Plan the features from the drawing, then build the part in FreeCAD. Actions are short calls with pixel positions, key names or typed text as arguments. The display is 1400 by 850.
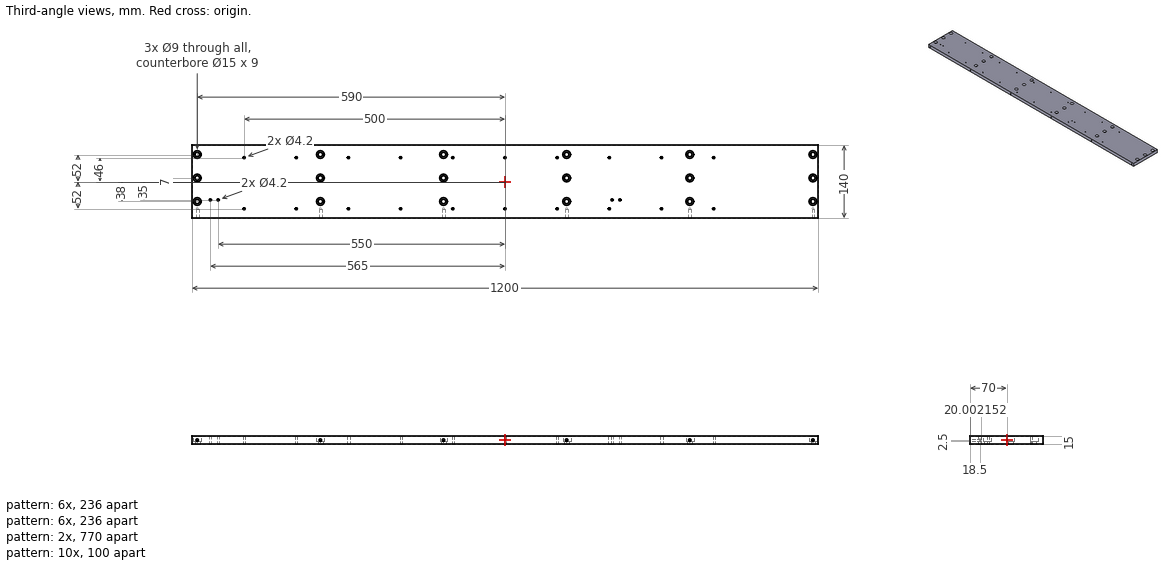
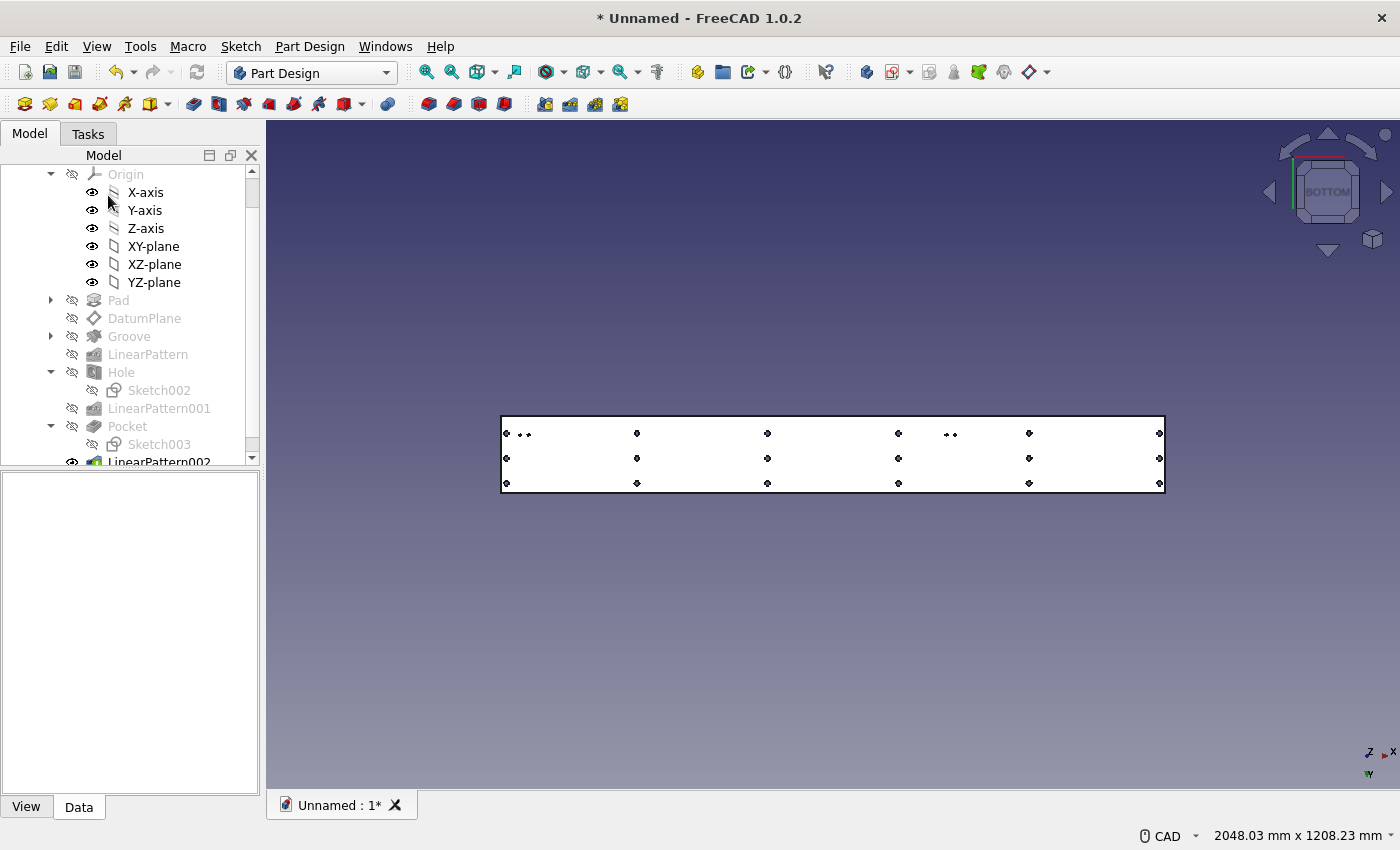
key(0)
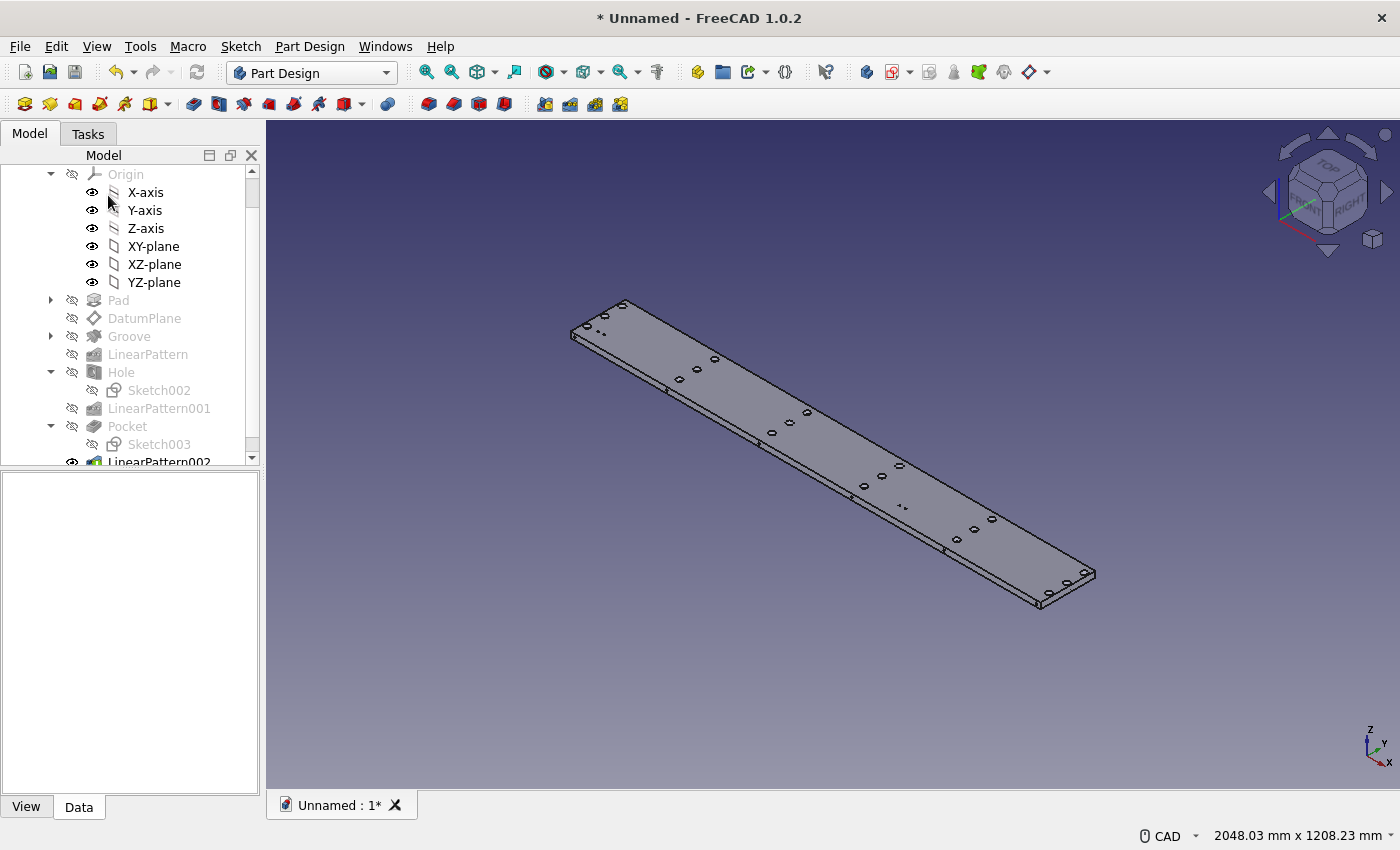
click(833, 450)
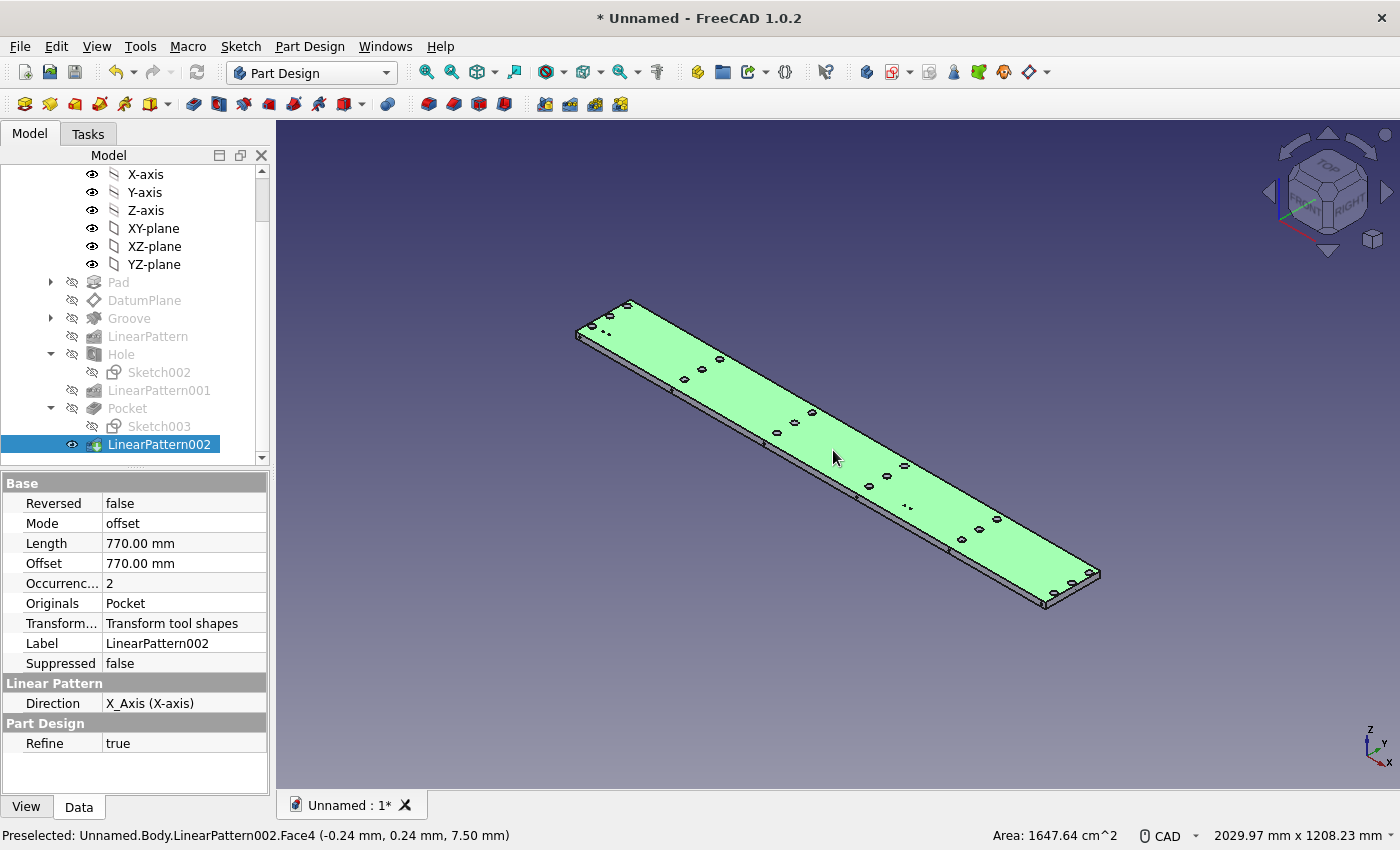
click(892, 72)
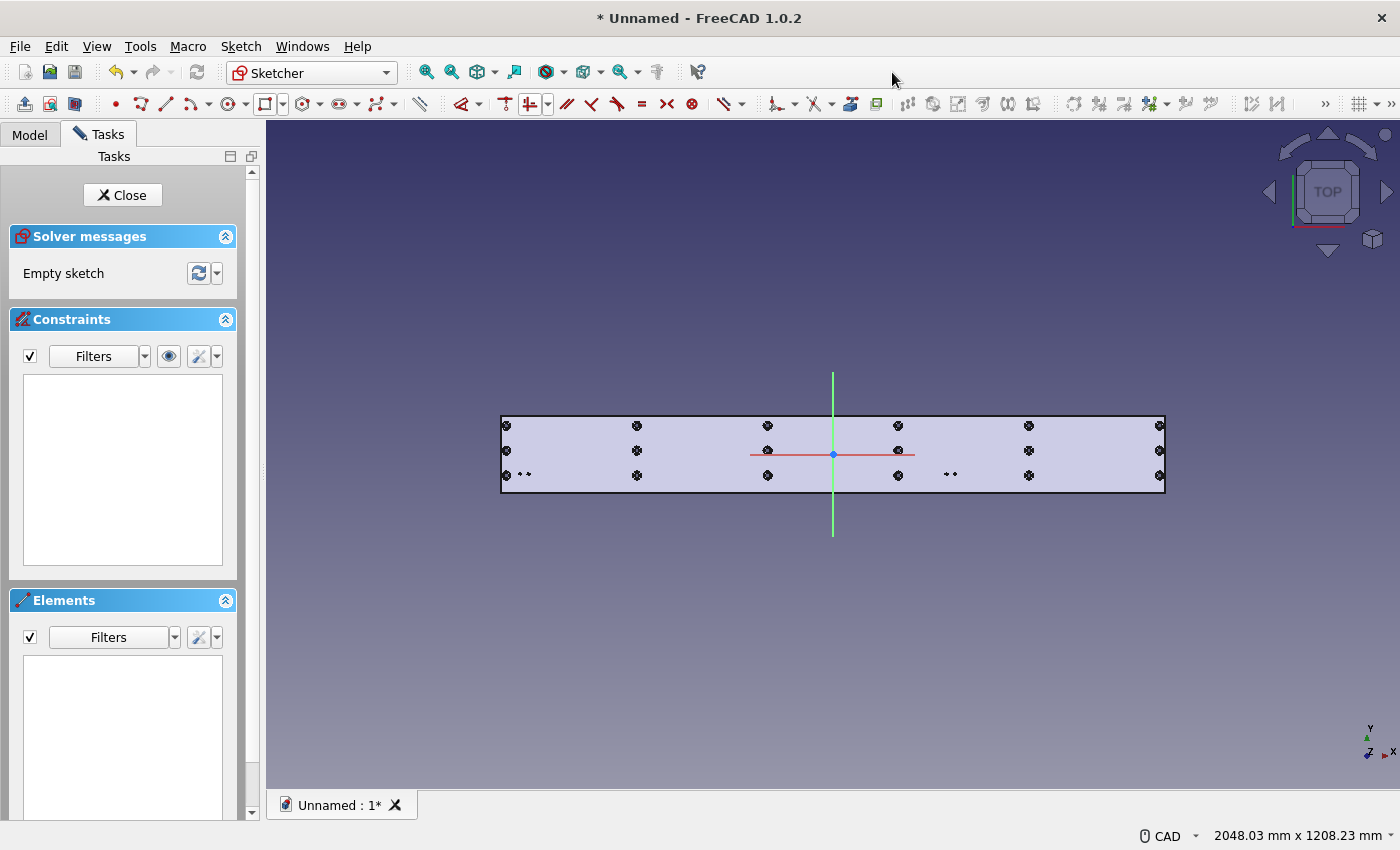
scroll(524, 456, up, 10)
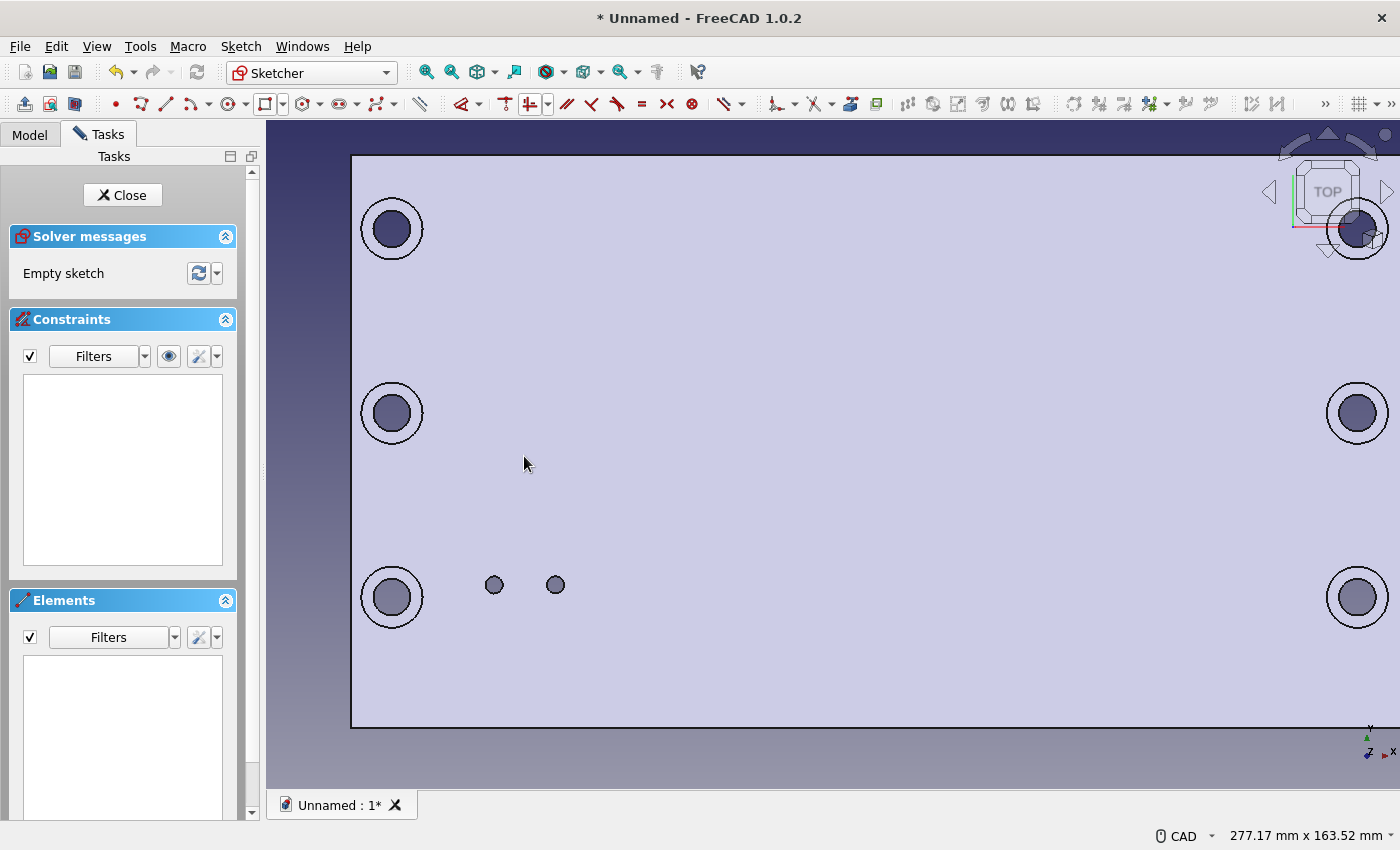
key(g)
key(c)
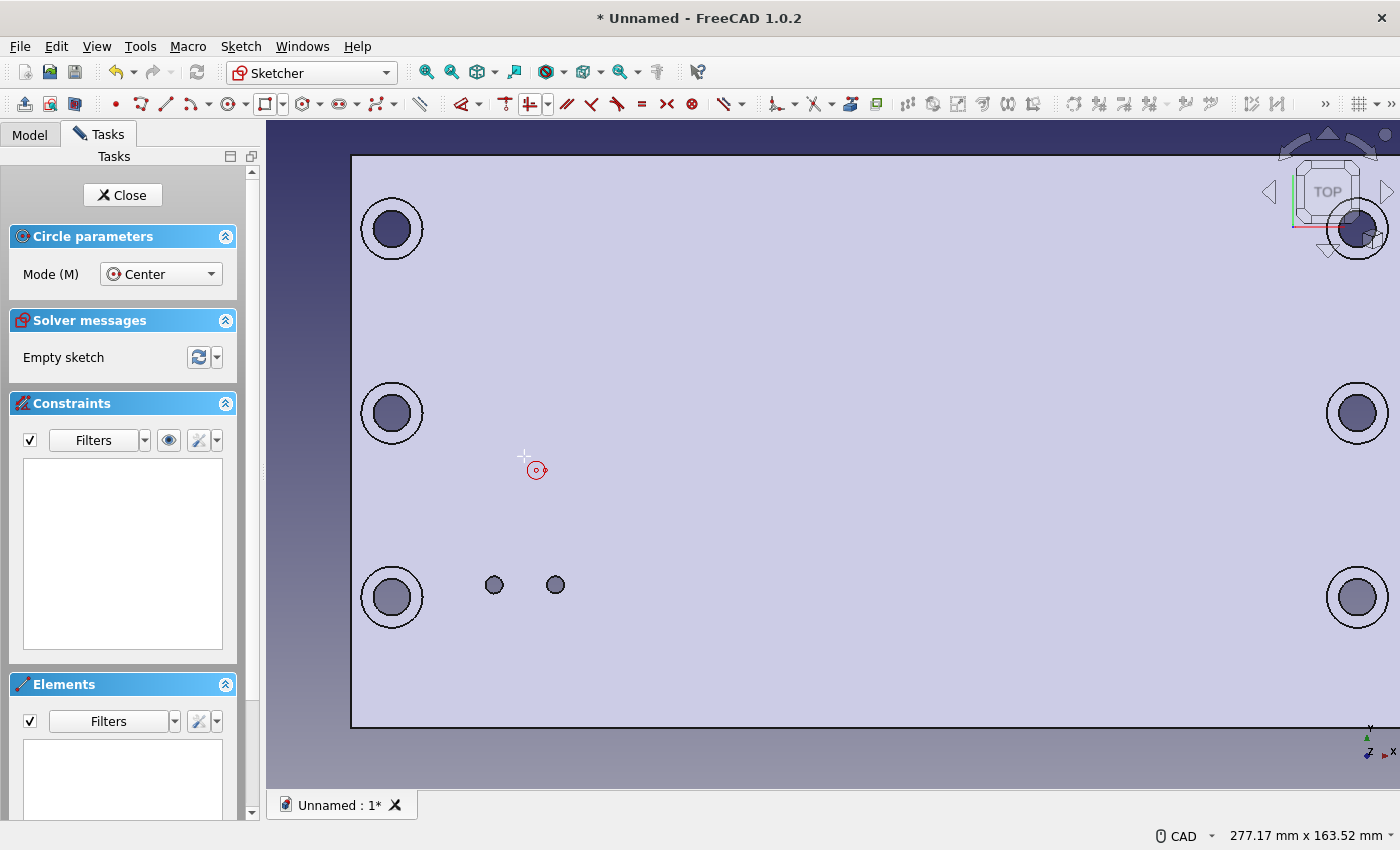
scroll(760, 254, up, 5)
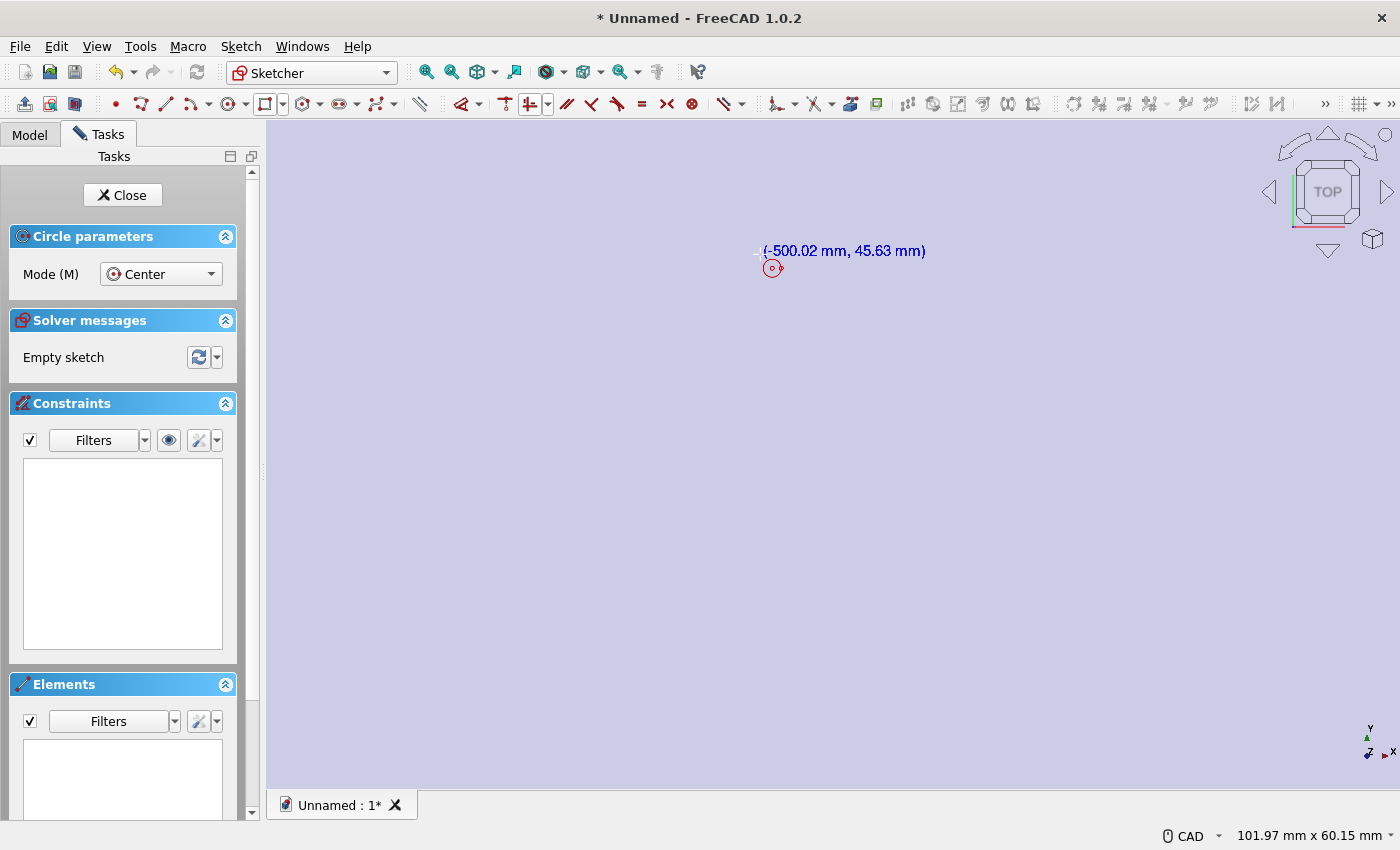
click(760, 252)
move(776, 236)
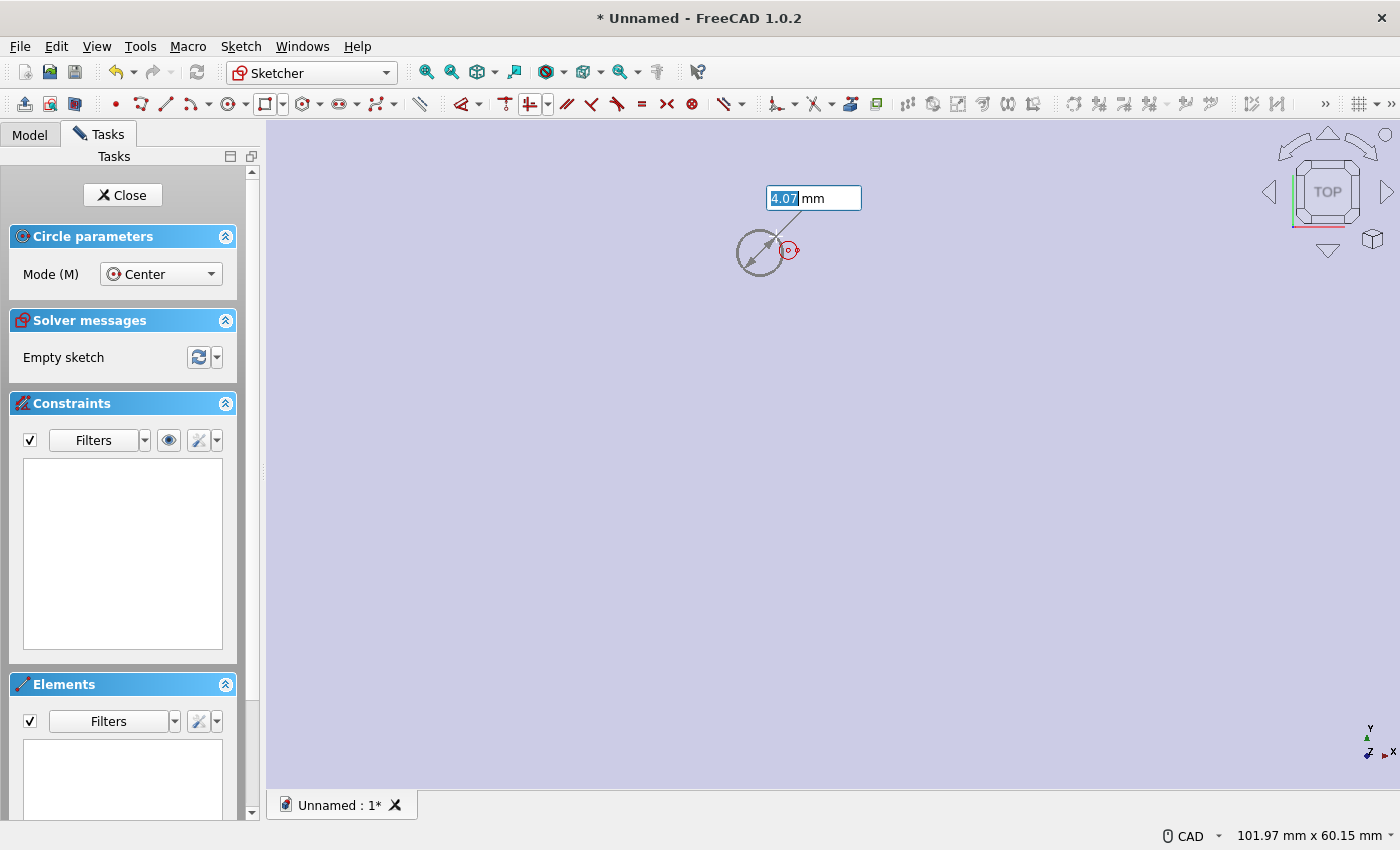
text(4.2)
key(Return)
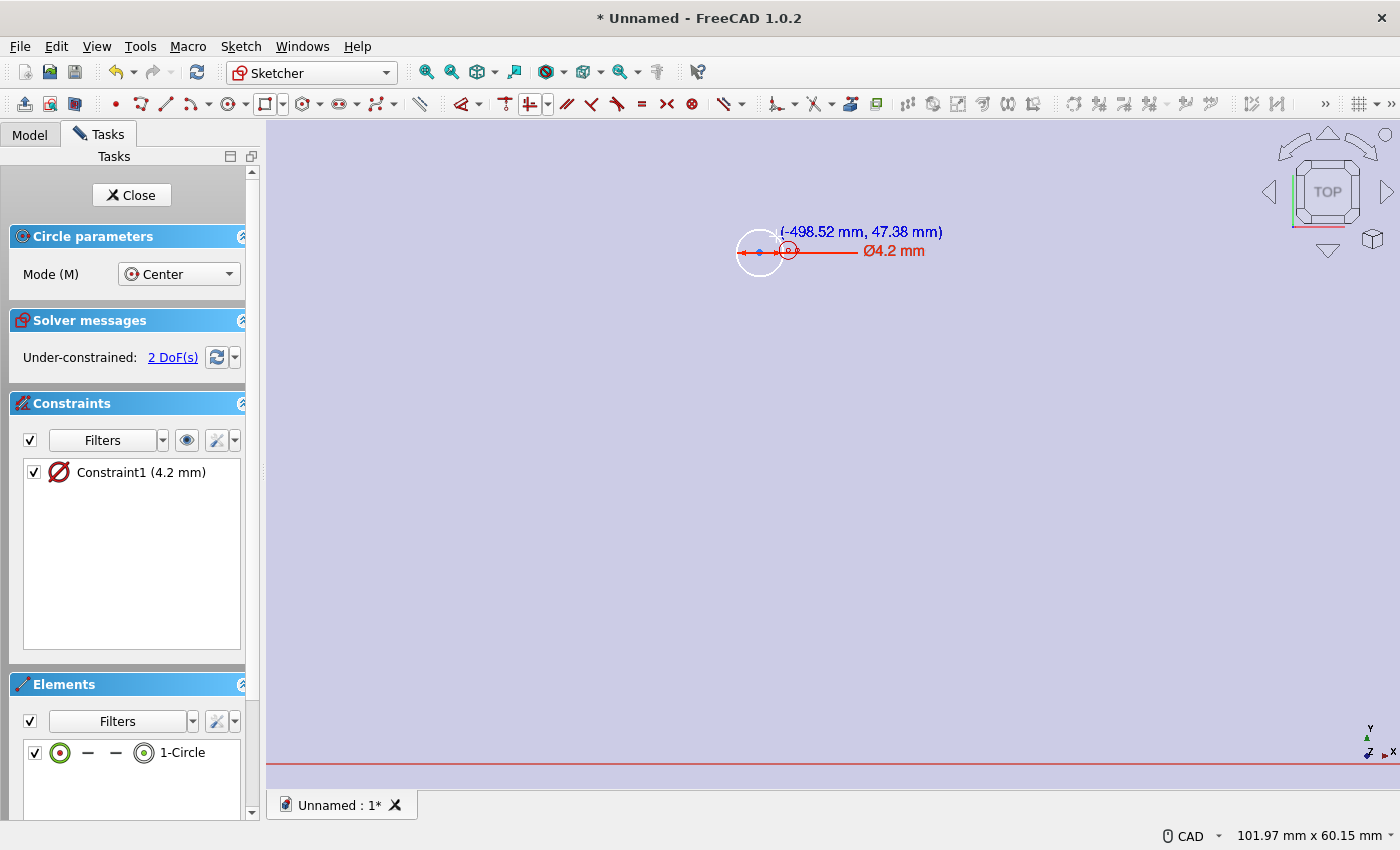
scroll(767, 255, down, 5)